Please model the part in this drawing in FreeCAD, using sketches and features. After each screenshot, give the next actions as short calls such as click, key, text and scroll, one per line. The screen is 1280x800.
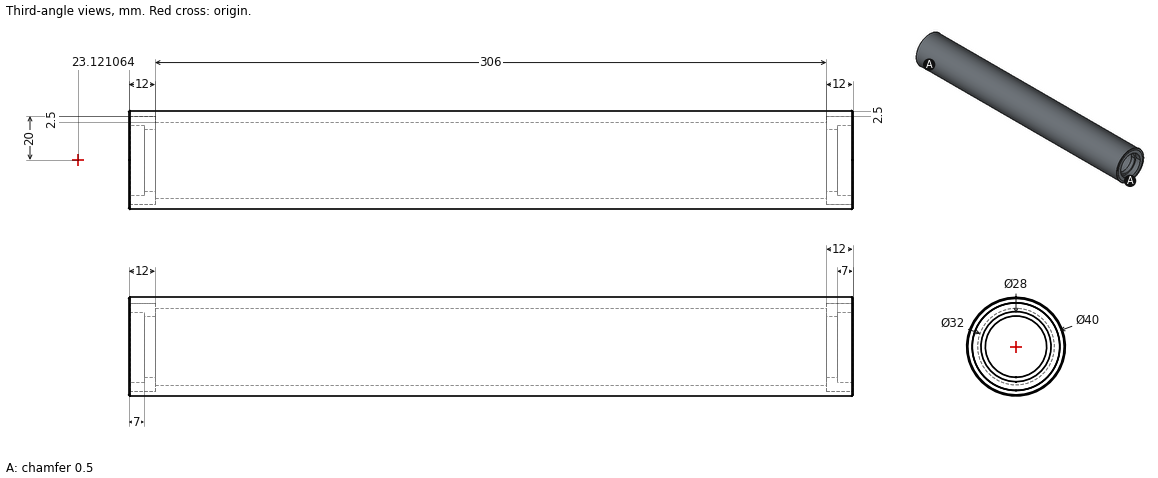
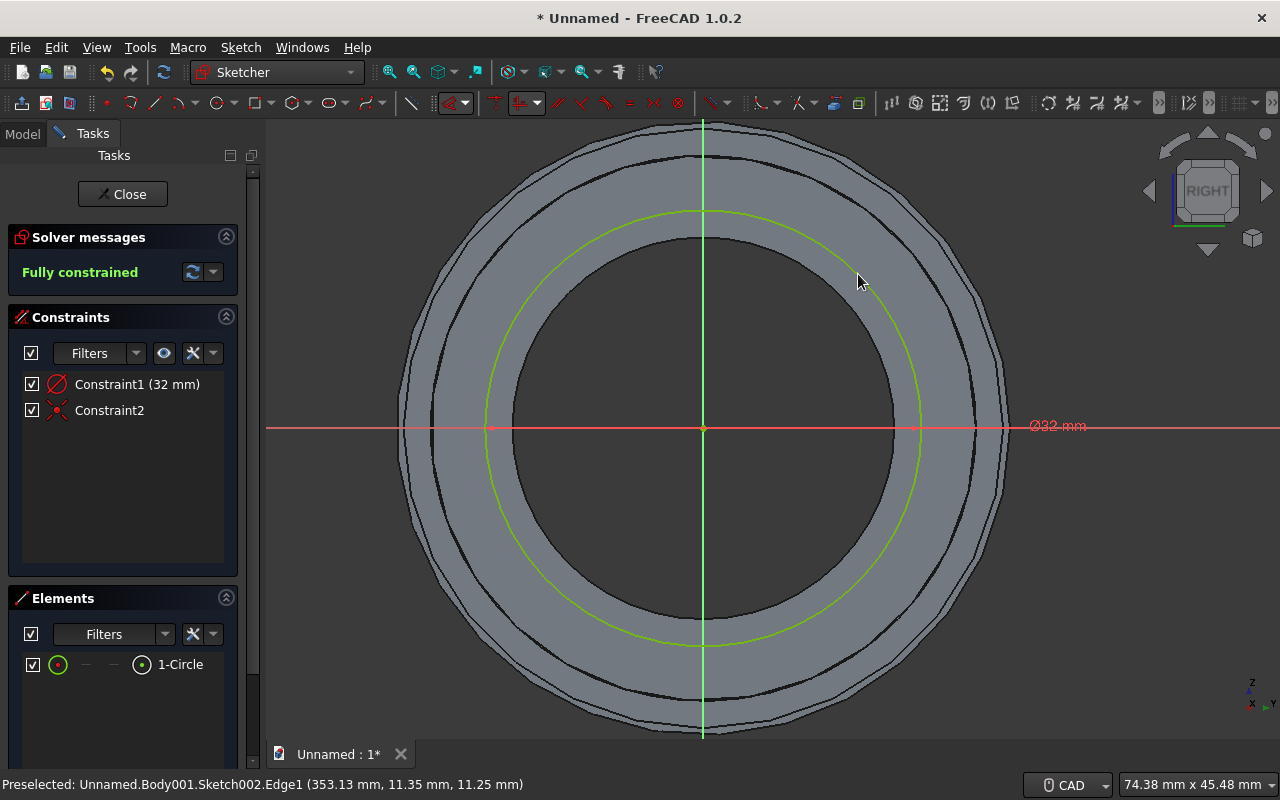
click(123, 194)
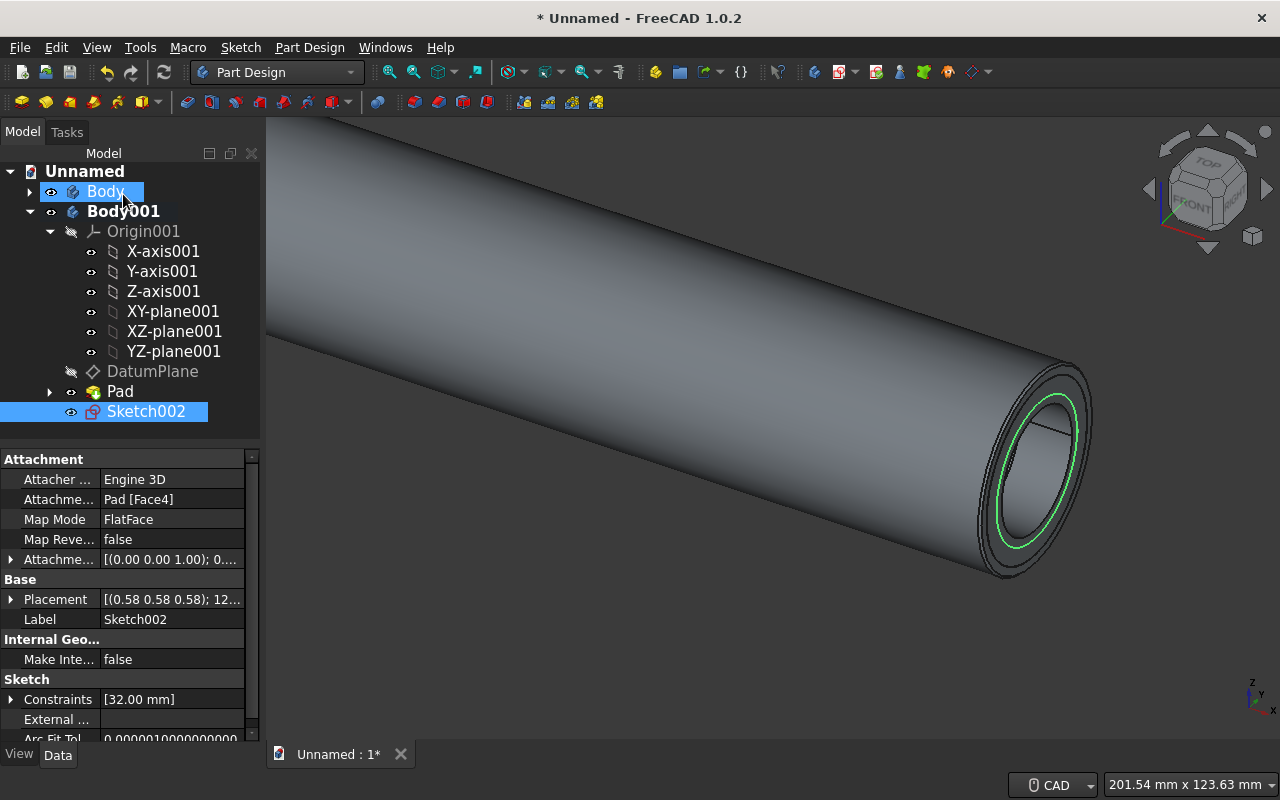
click(188, 102)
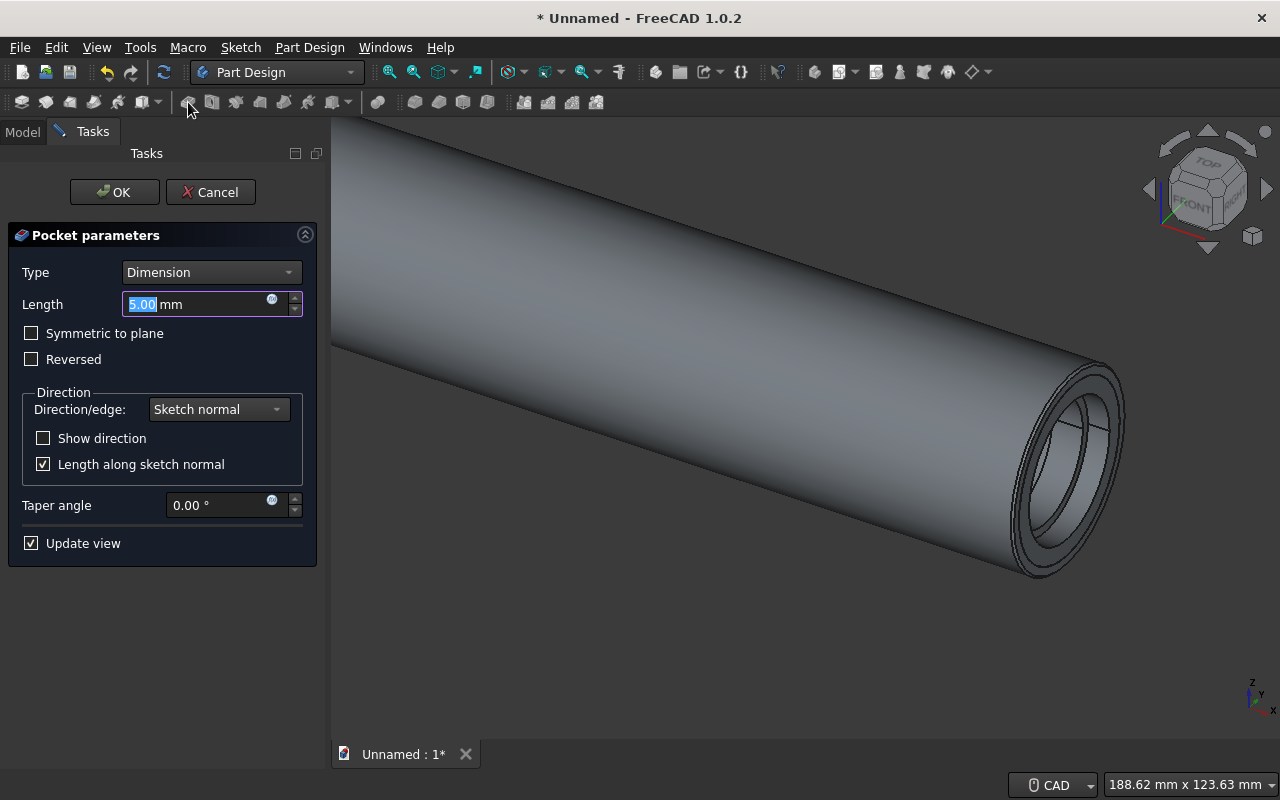
text(7)
key(Tab)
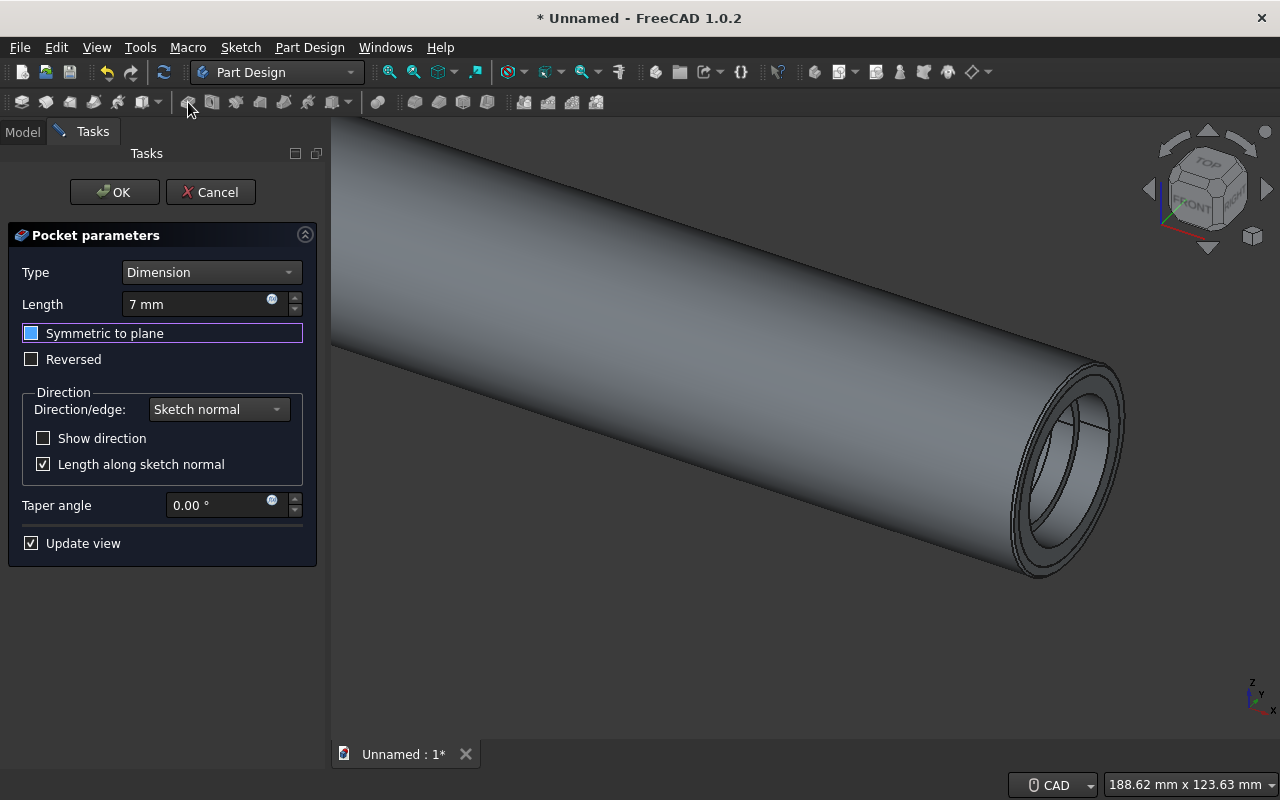
click(115, 192)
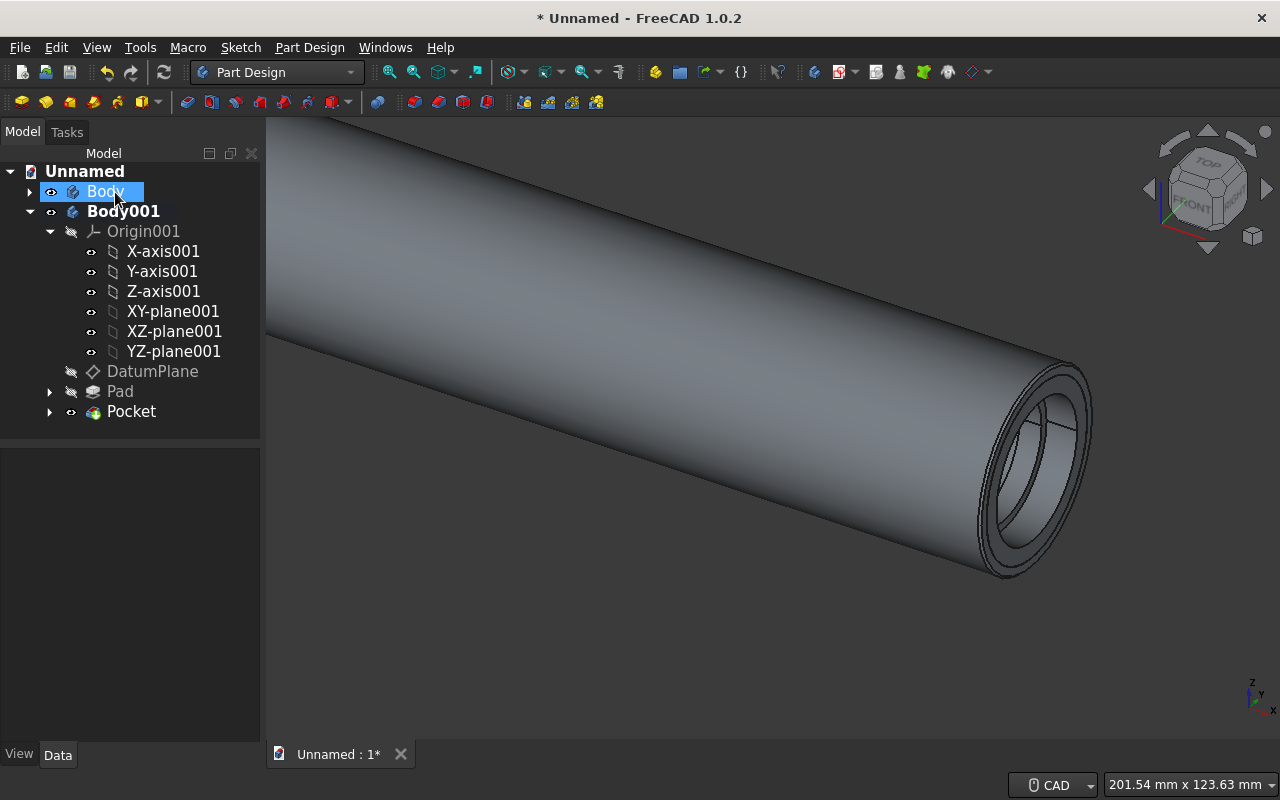
click(816, 72)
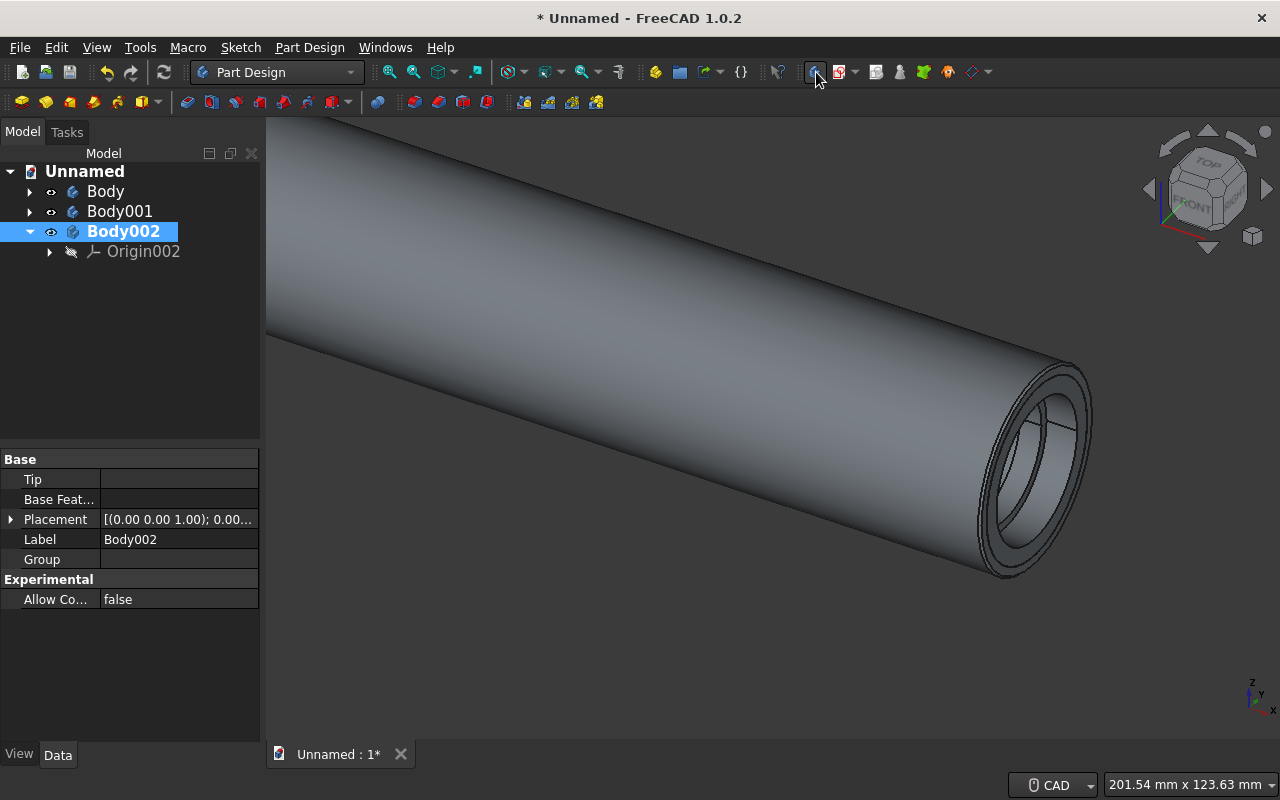
click(50, 252)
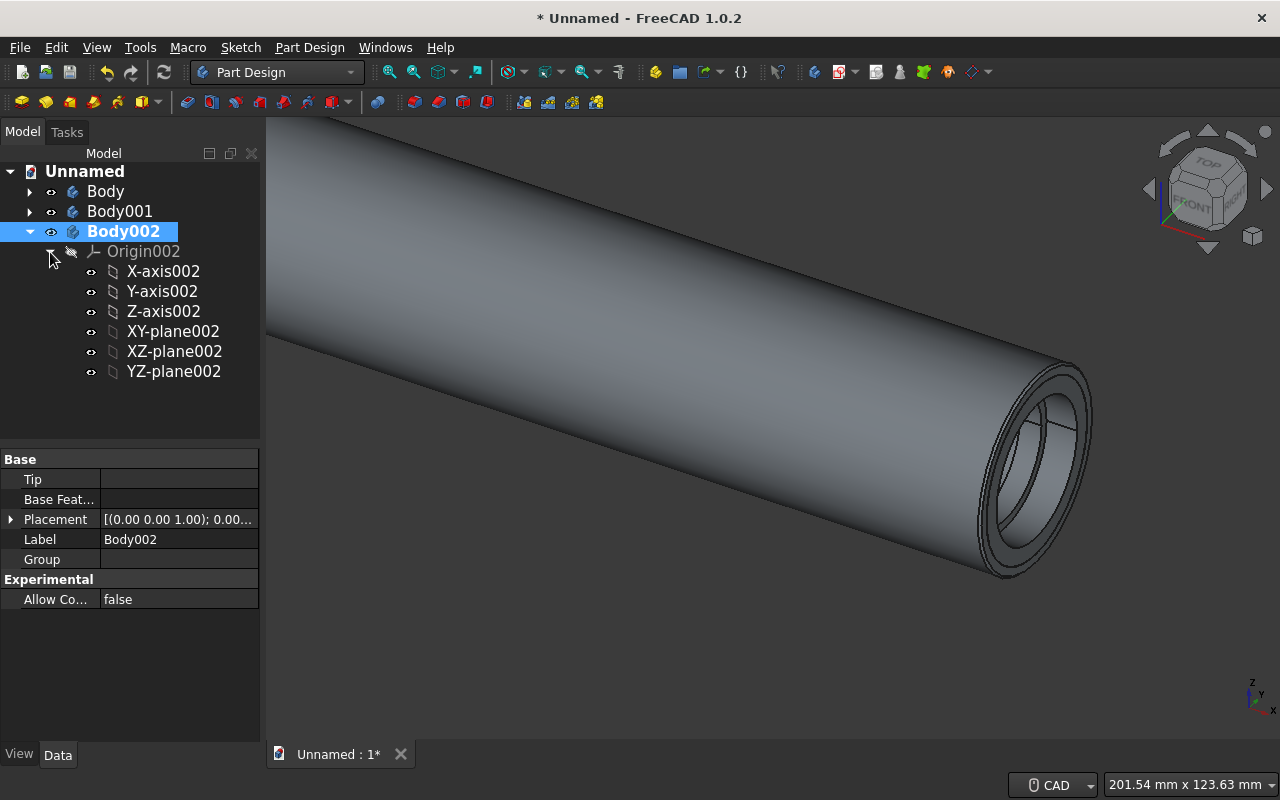
click(136, 372)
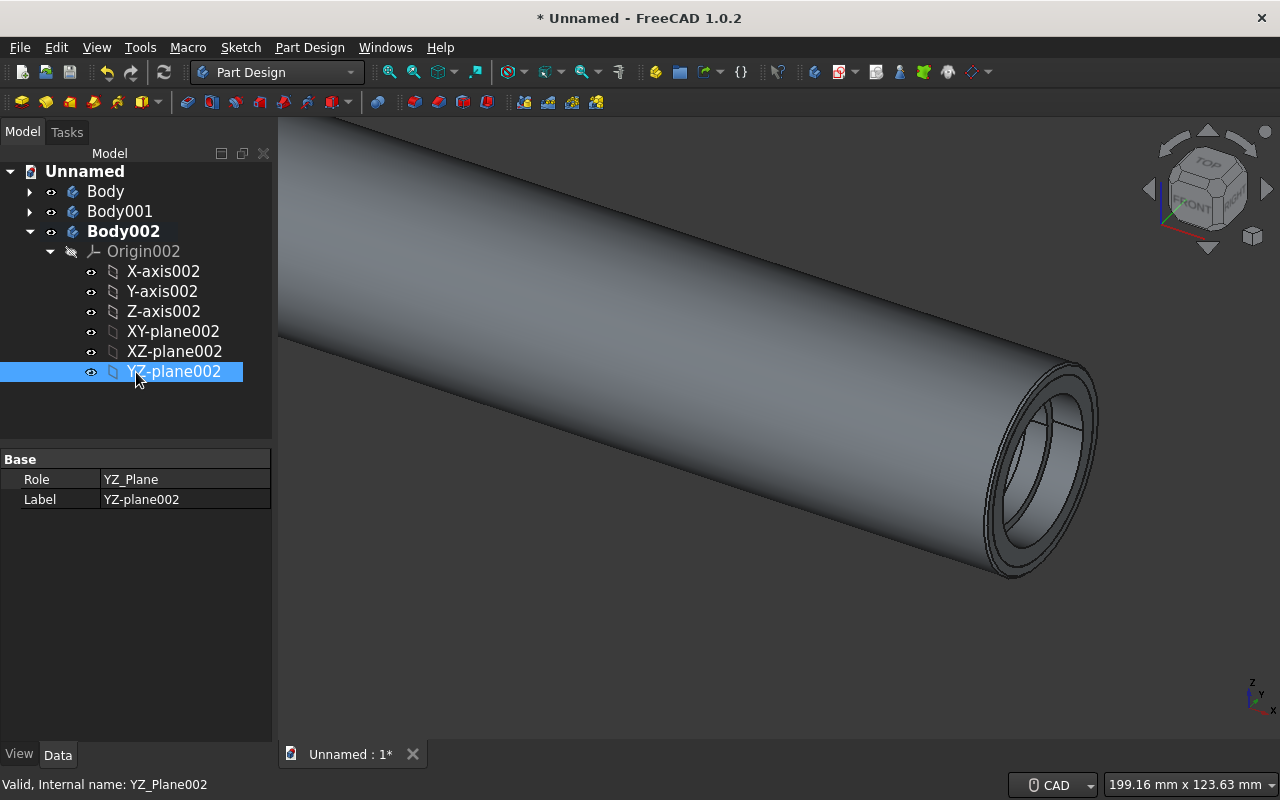
click(972, 72)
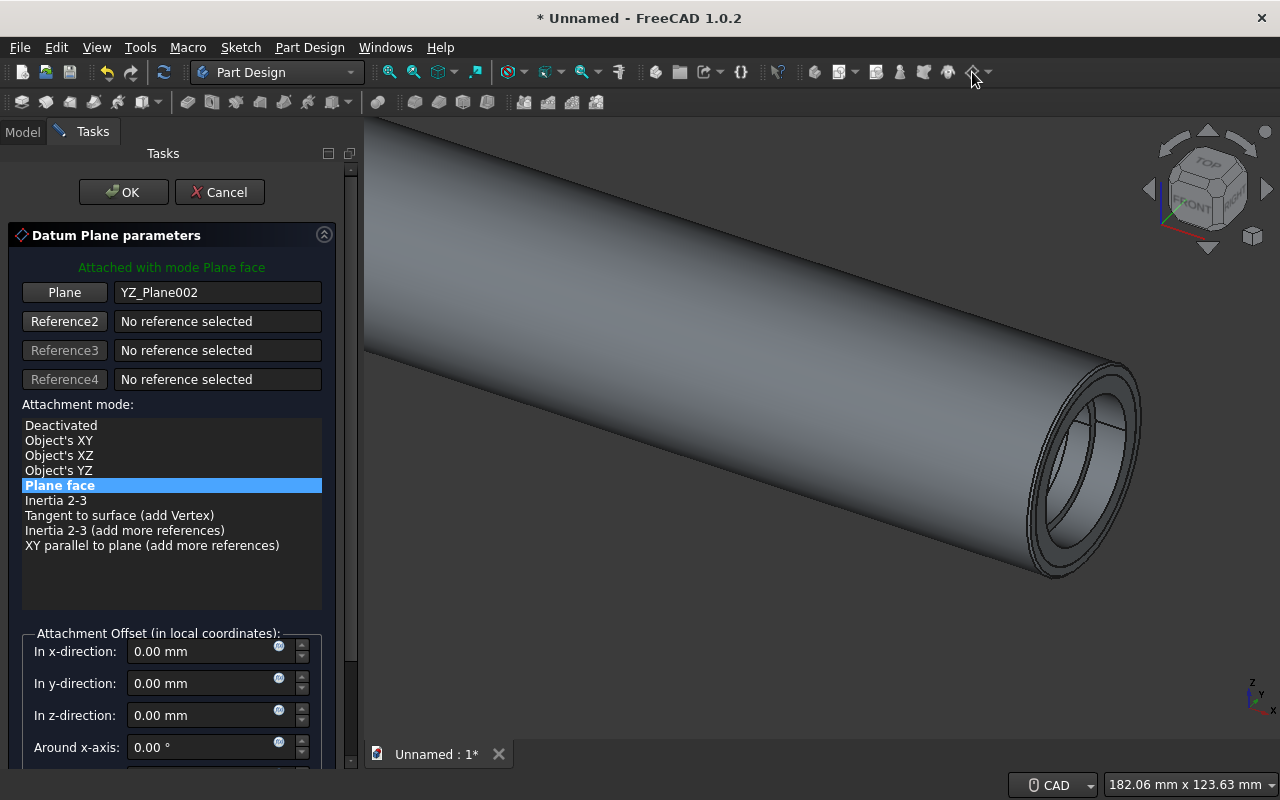
triple_click(210, 715)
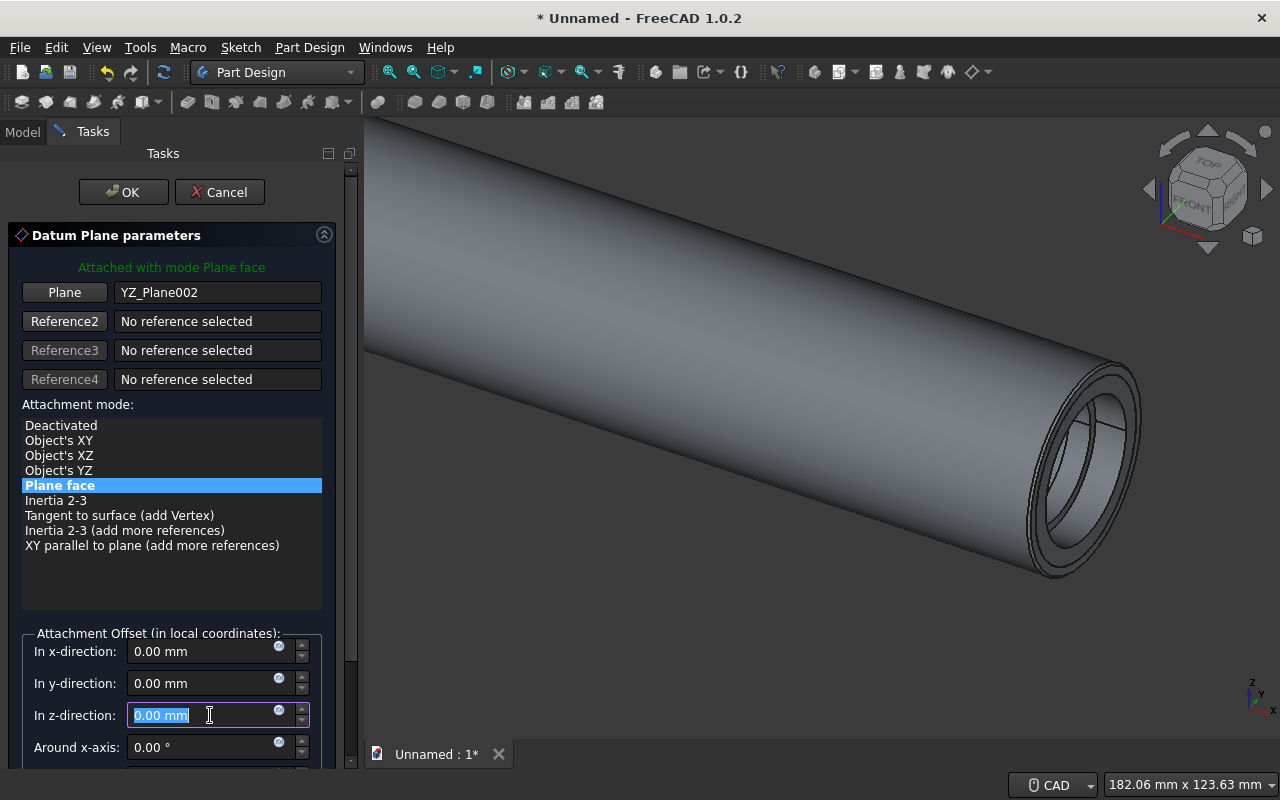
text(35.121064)
key(Tab)